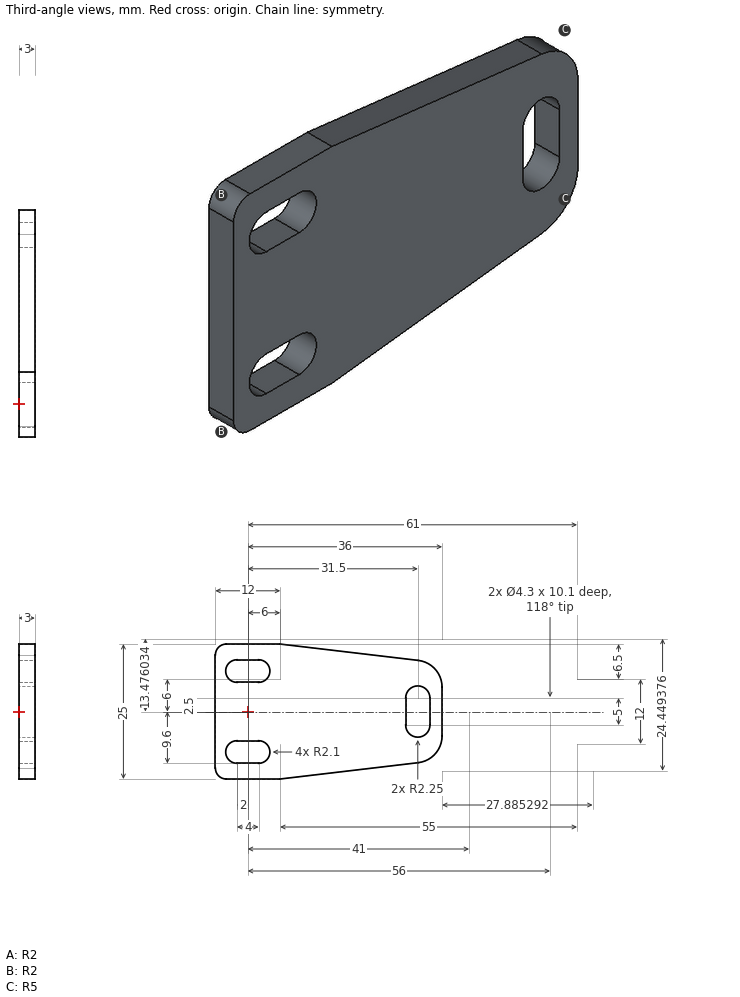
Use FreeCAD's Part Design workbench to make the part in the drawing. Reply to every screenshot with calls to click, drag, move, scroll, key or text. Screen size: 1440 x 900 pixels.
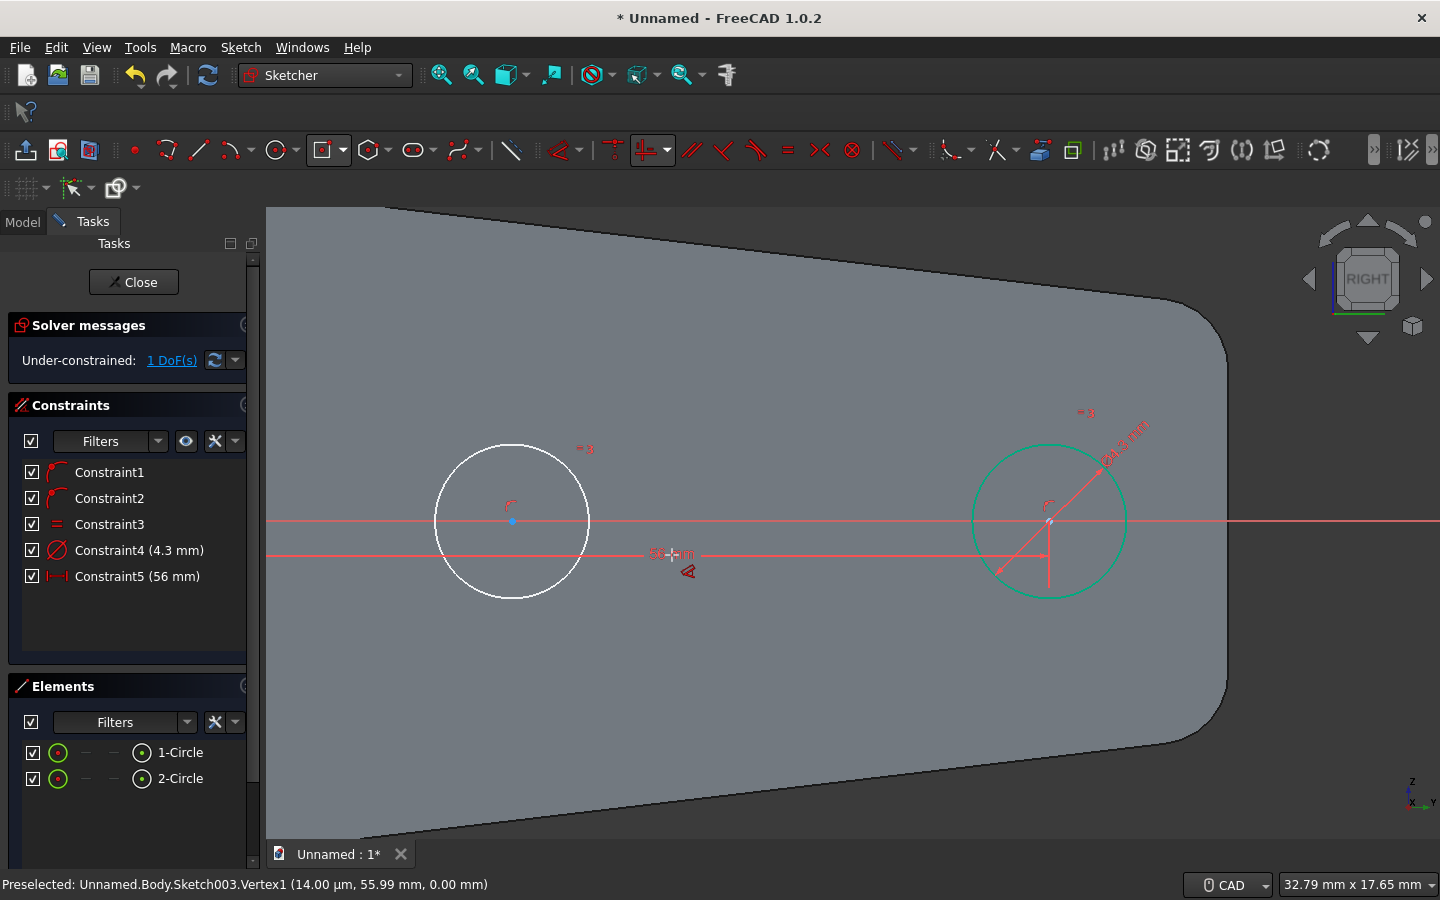
click(512, 521)
click(403, 555)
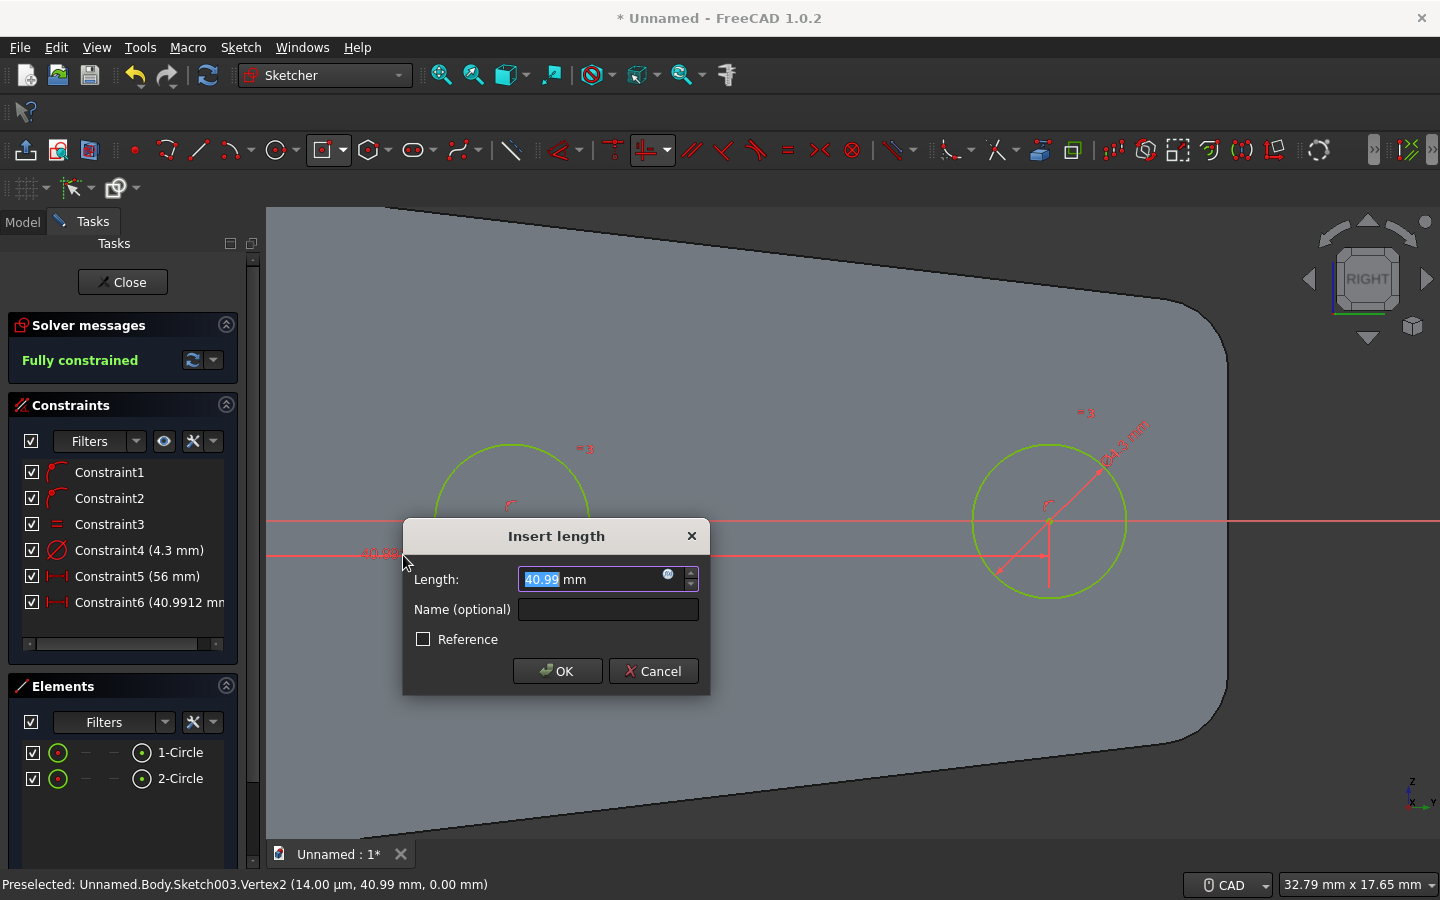
text(41)
key(Return)
key(Escape)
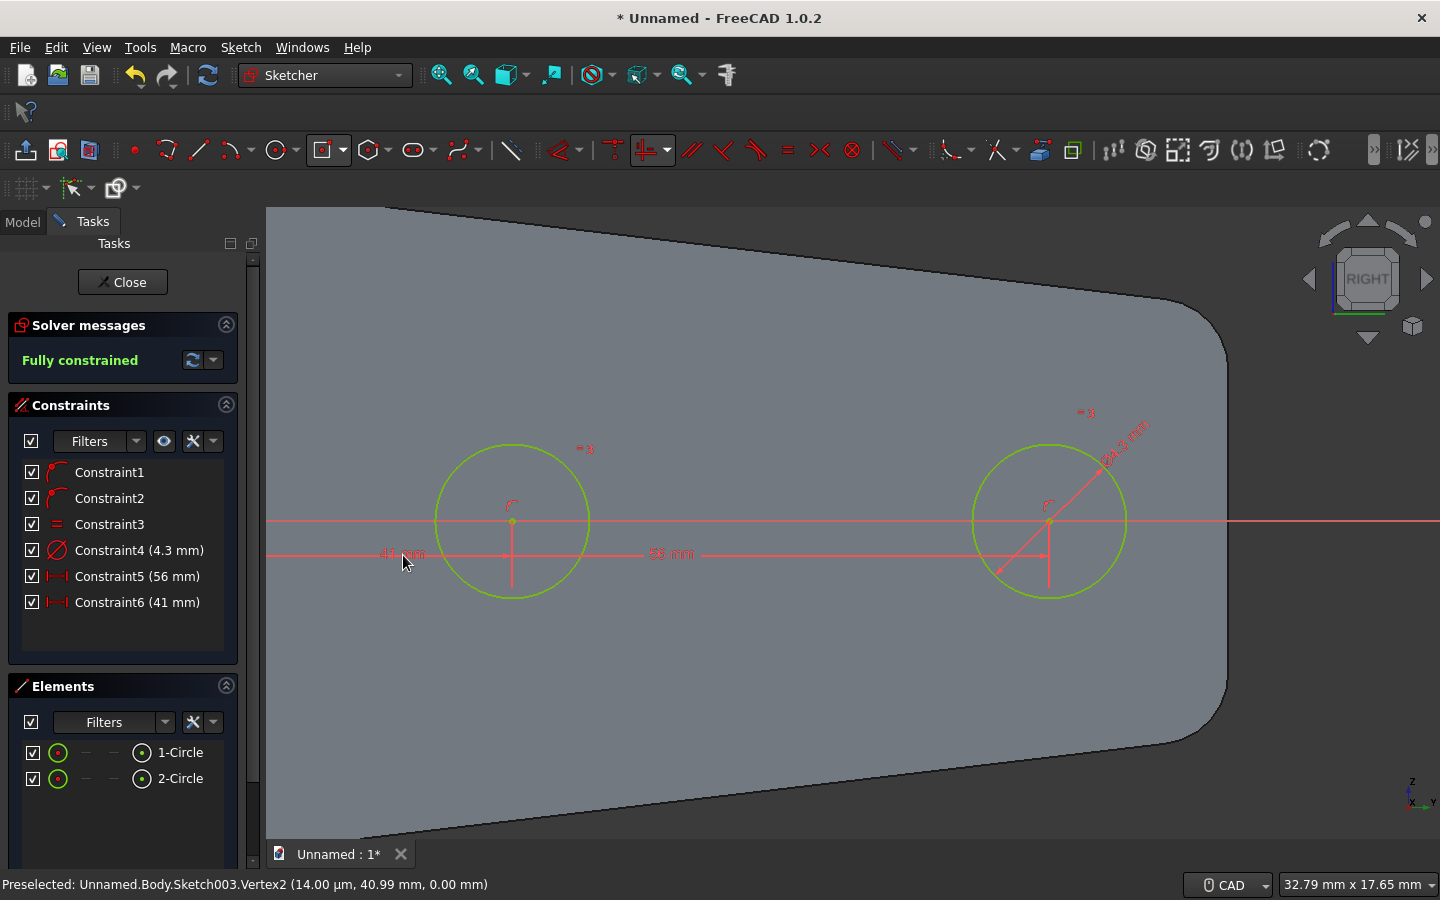
click(123, 282)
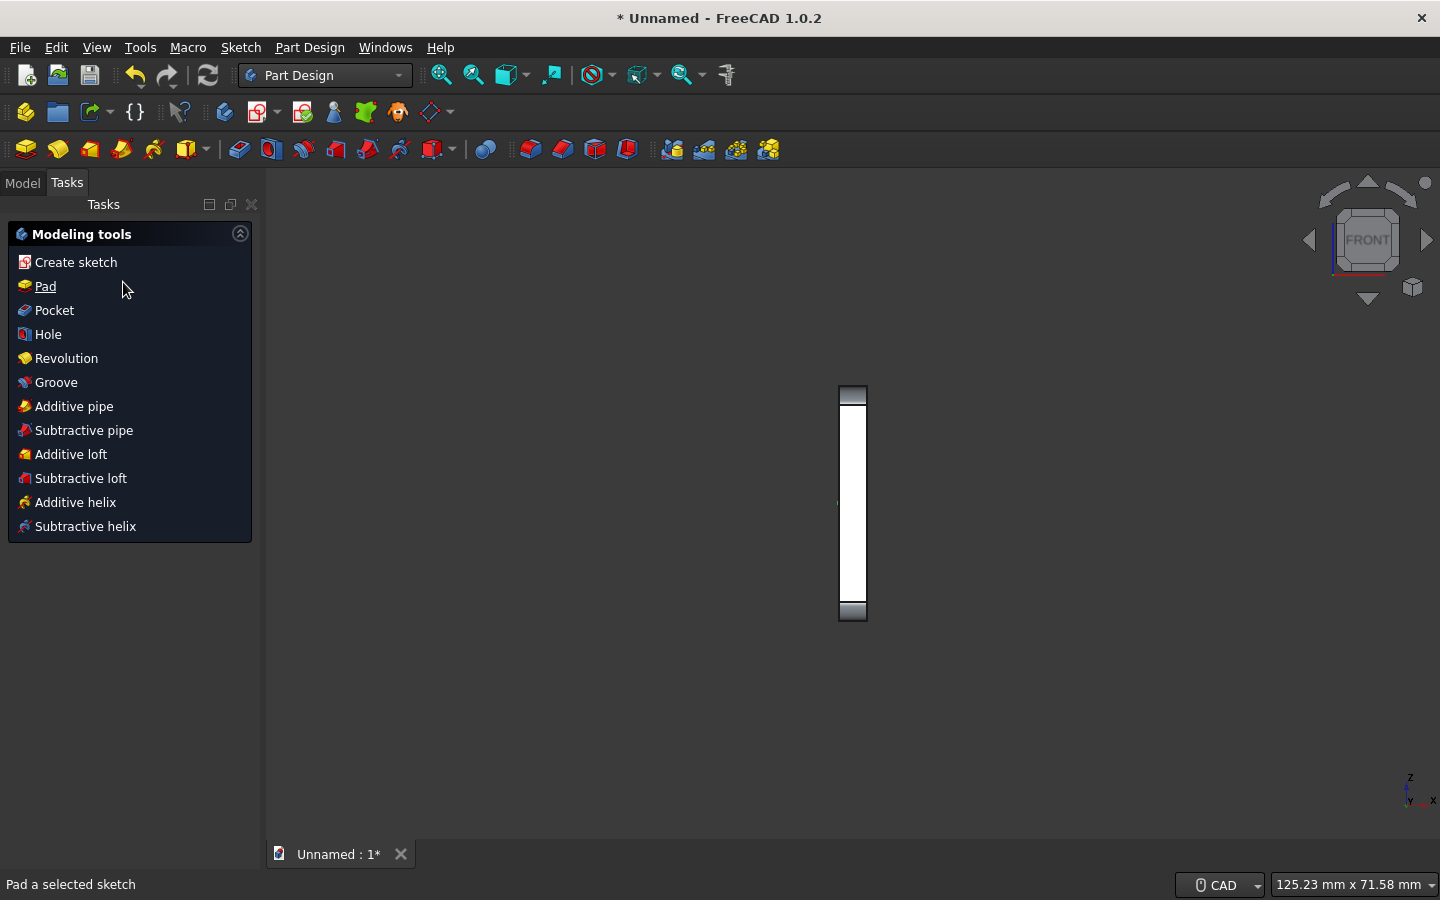
click(272, 150)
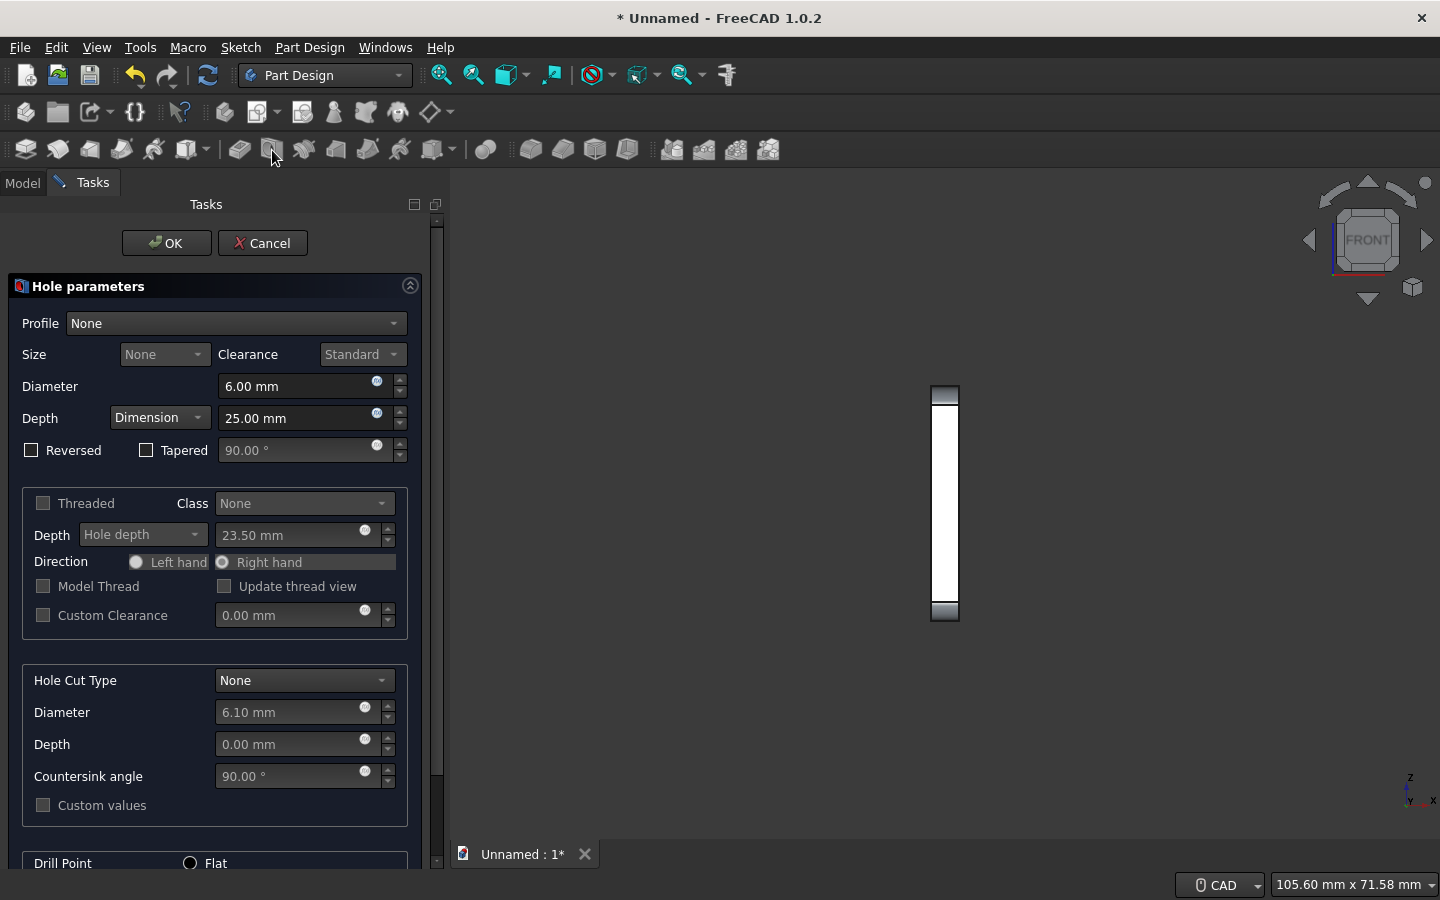
triple_click(305, 386)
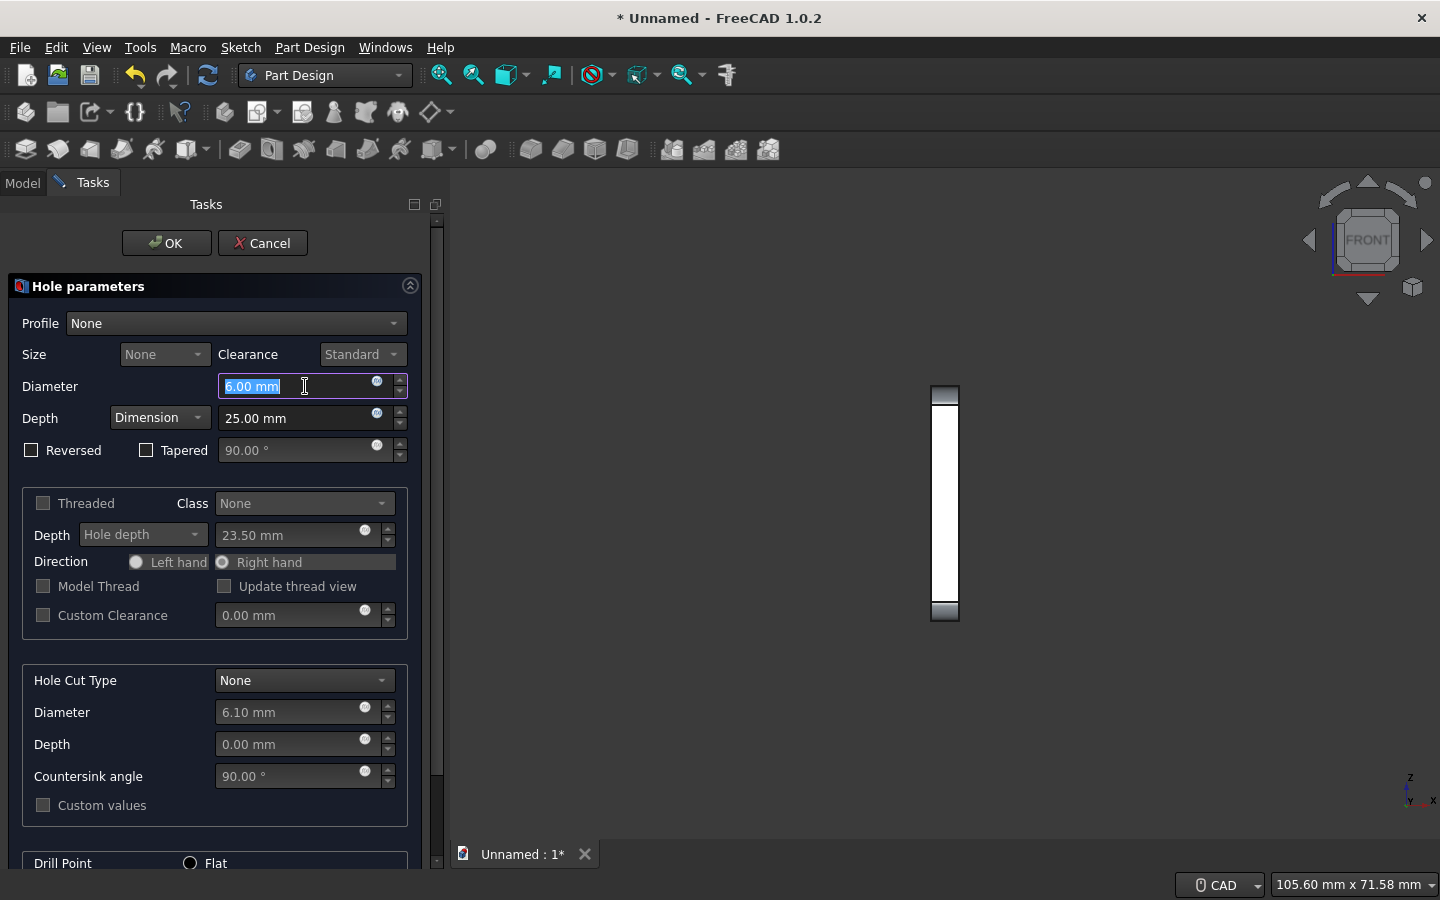
text(4.3)
key(Tab)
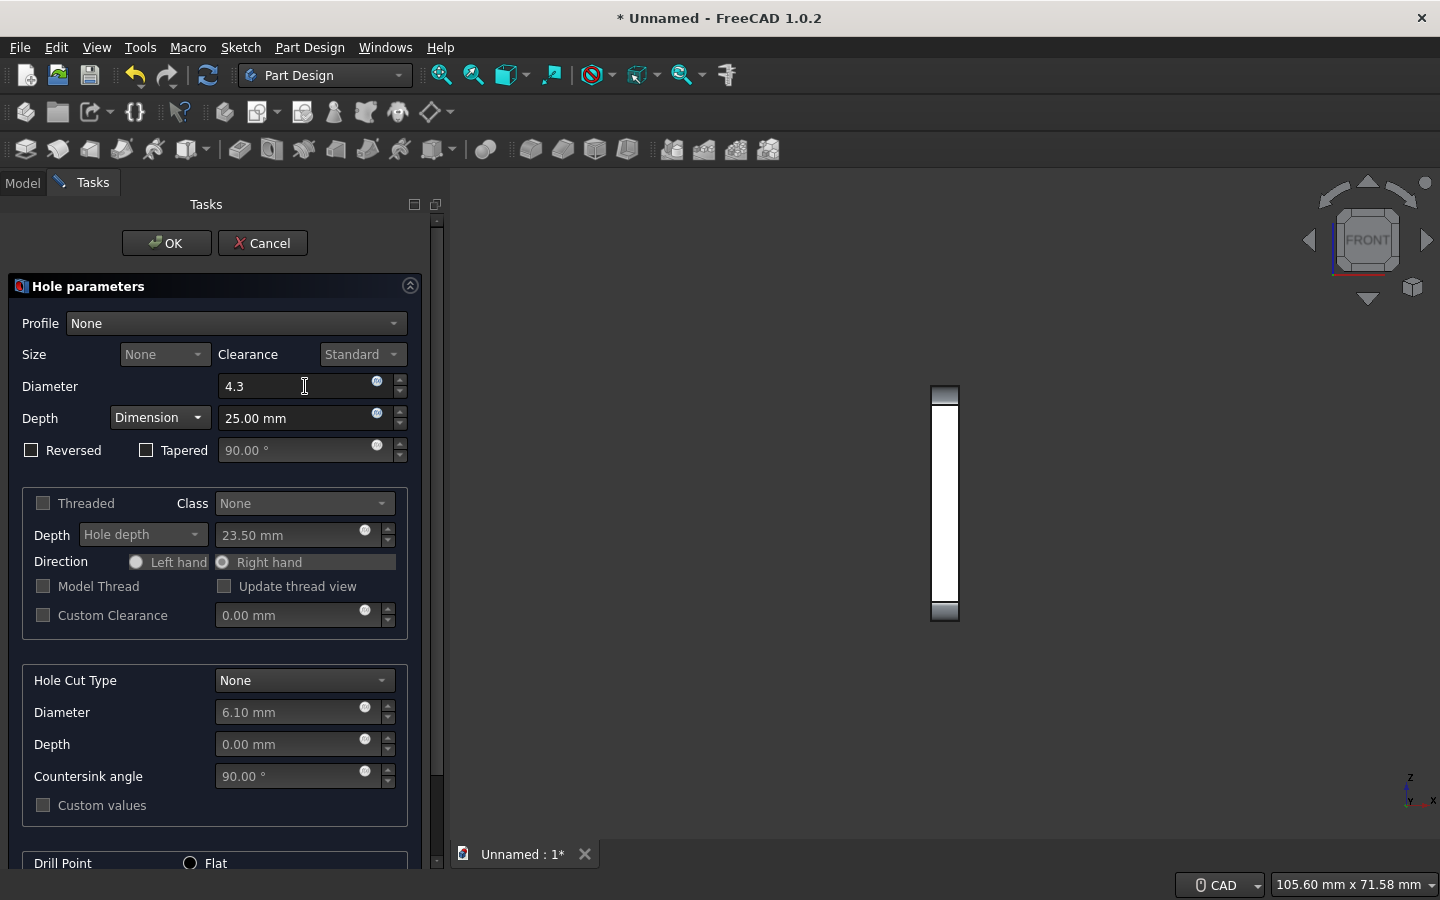
triple_click(305, 418)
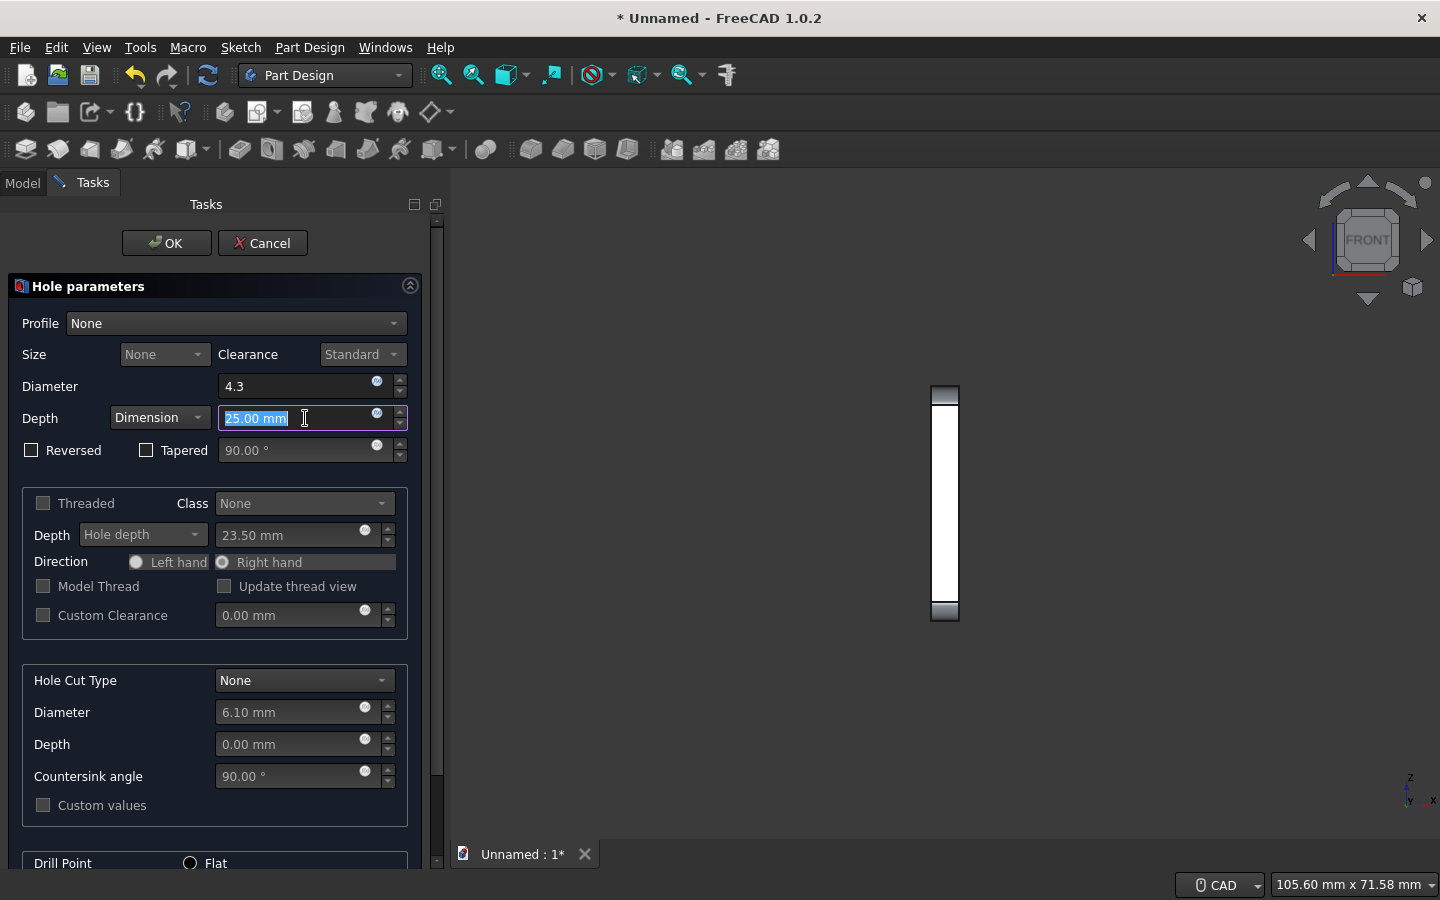
text(10.1)
key(Tab)